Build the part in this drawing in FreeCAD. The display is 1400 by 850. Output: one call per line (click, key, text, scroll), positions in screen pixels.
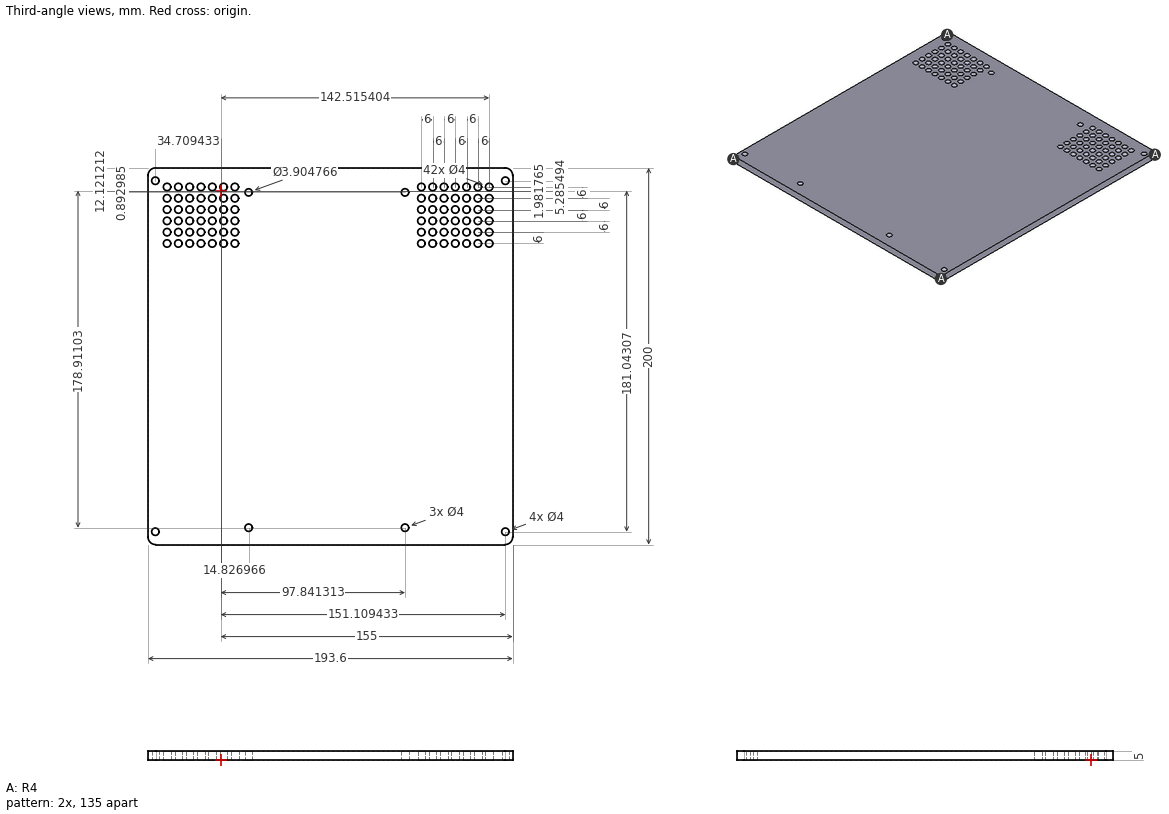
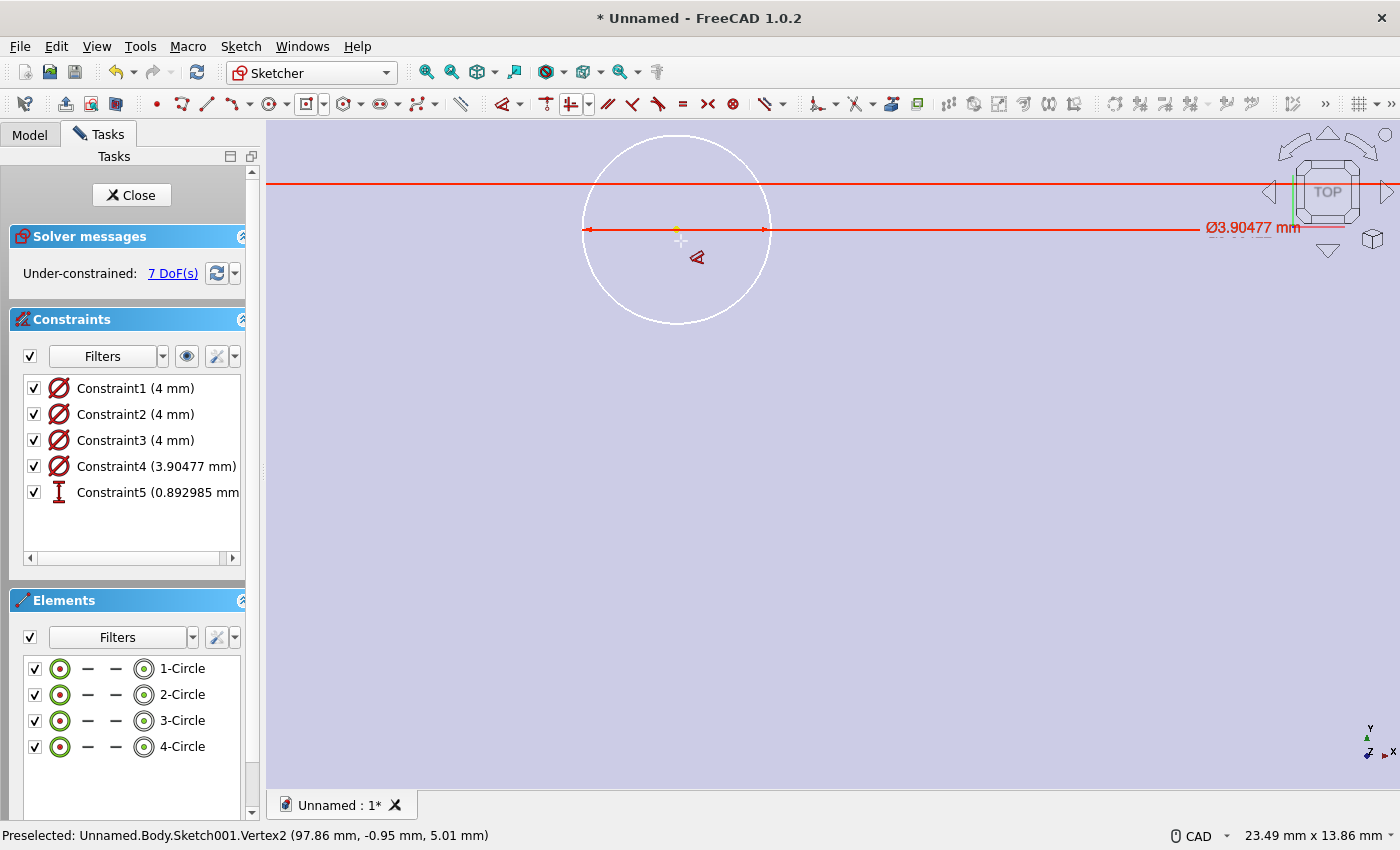
click(677, 230)
click(711, 207)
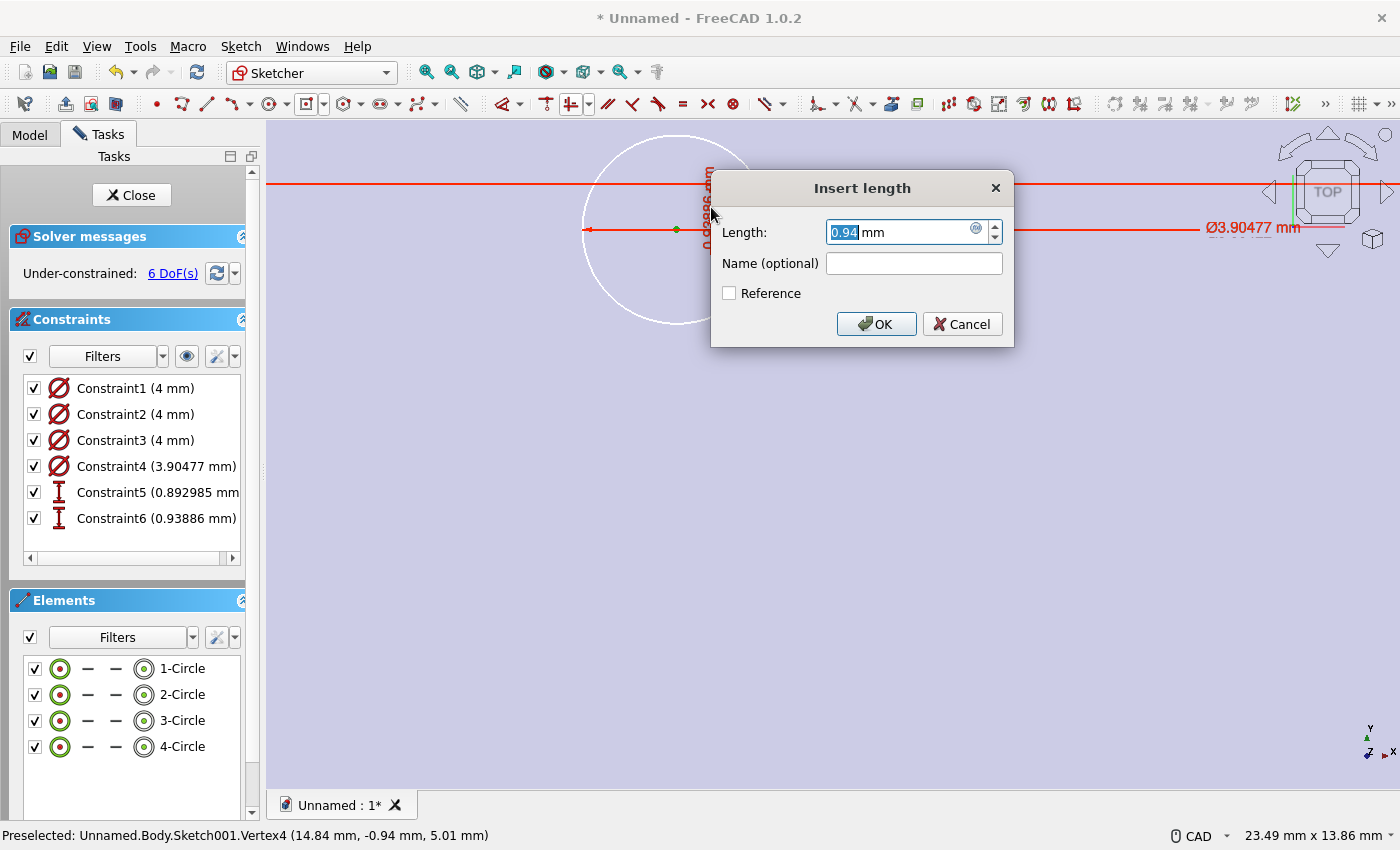
text(0.892985)
key(Return)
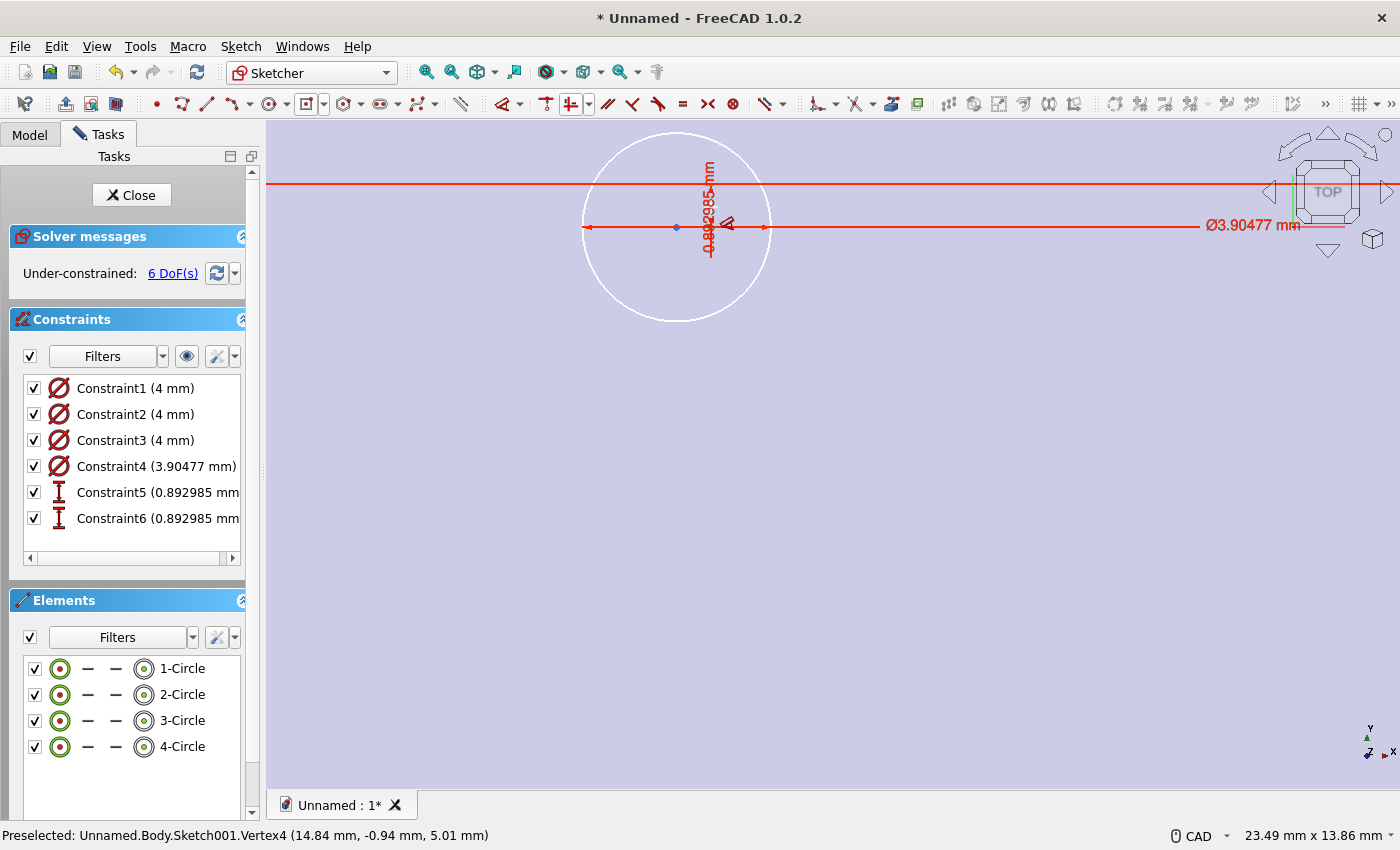
scroll(680, 241, down, 15)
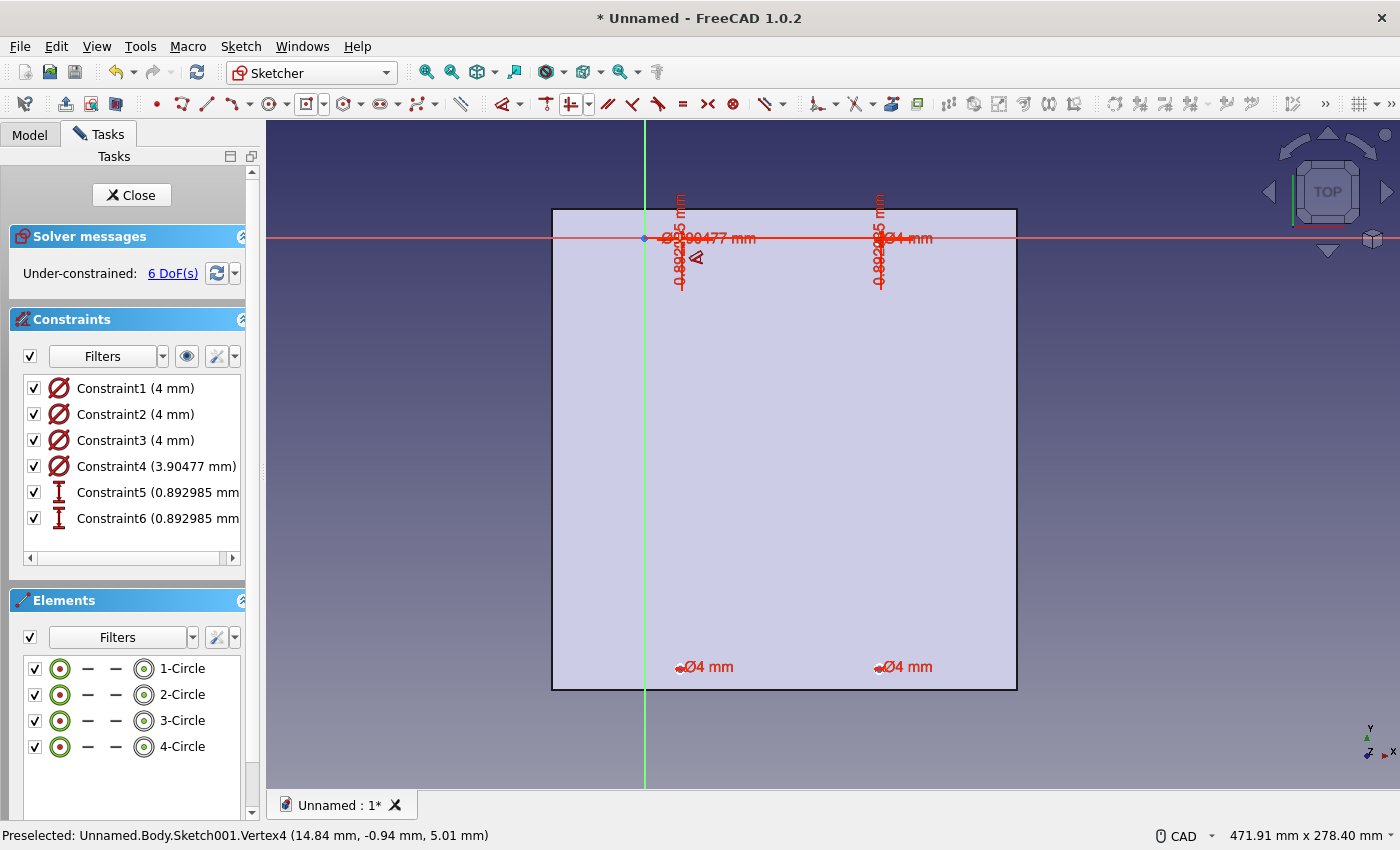
click(879, 669)
click(762, 204)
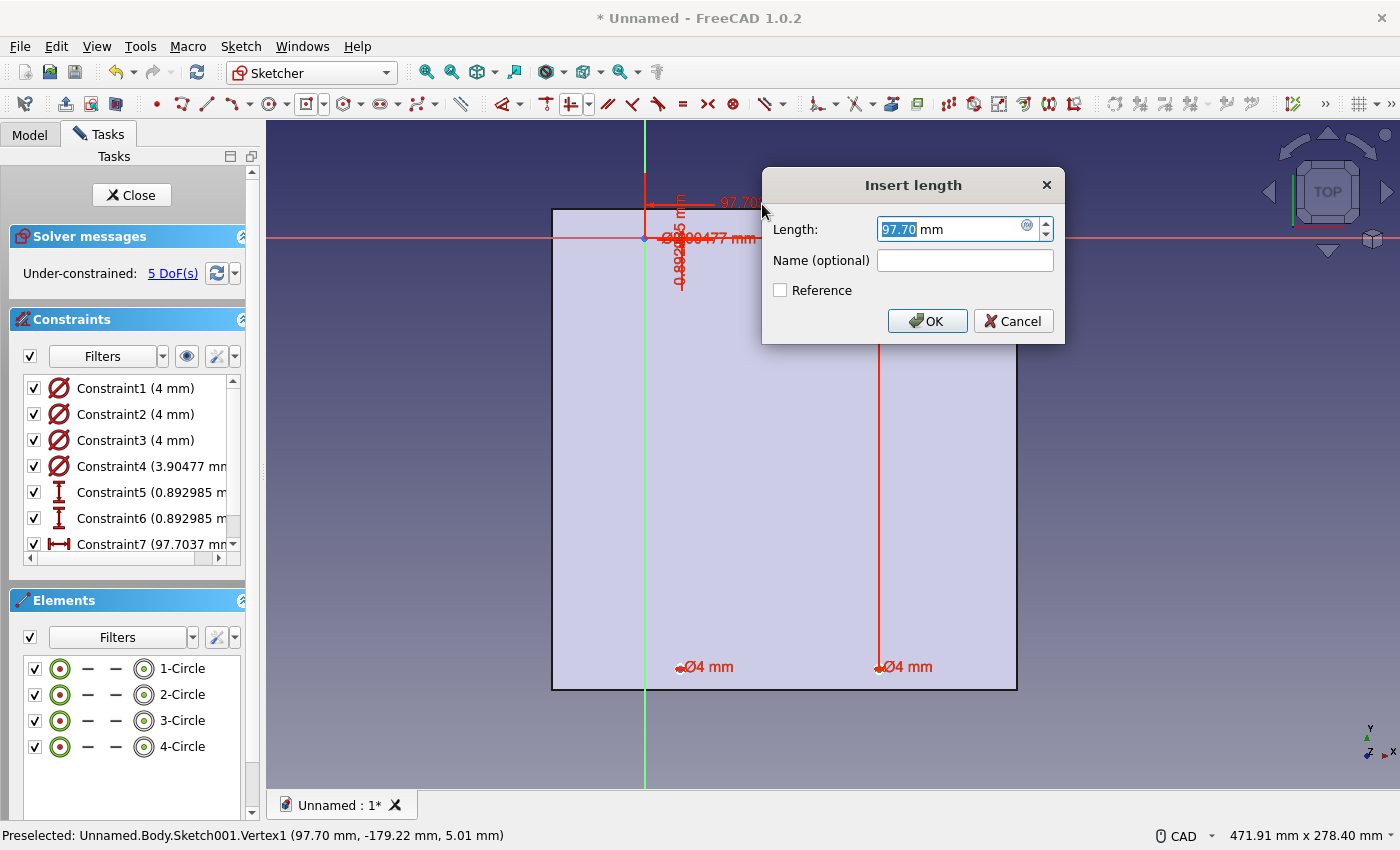
text(97.841313)
key(Return)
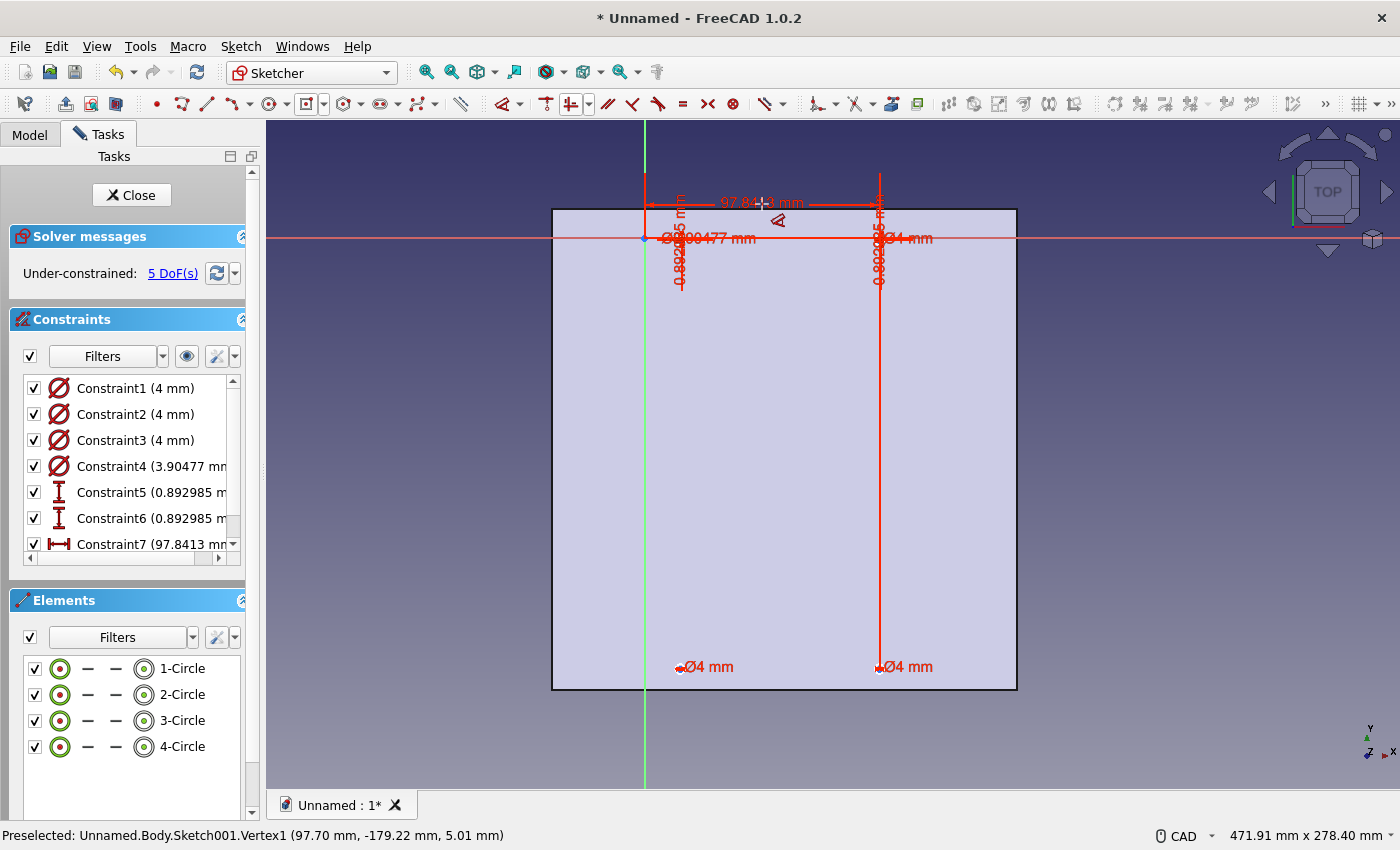
click(880, 669)
click(611, 454)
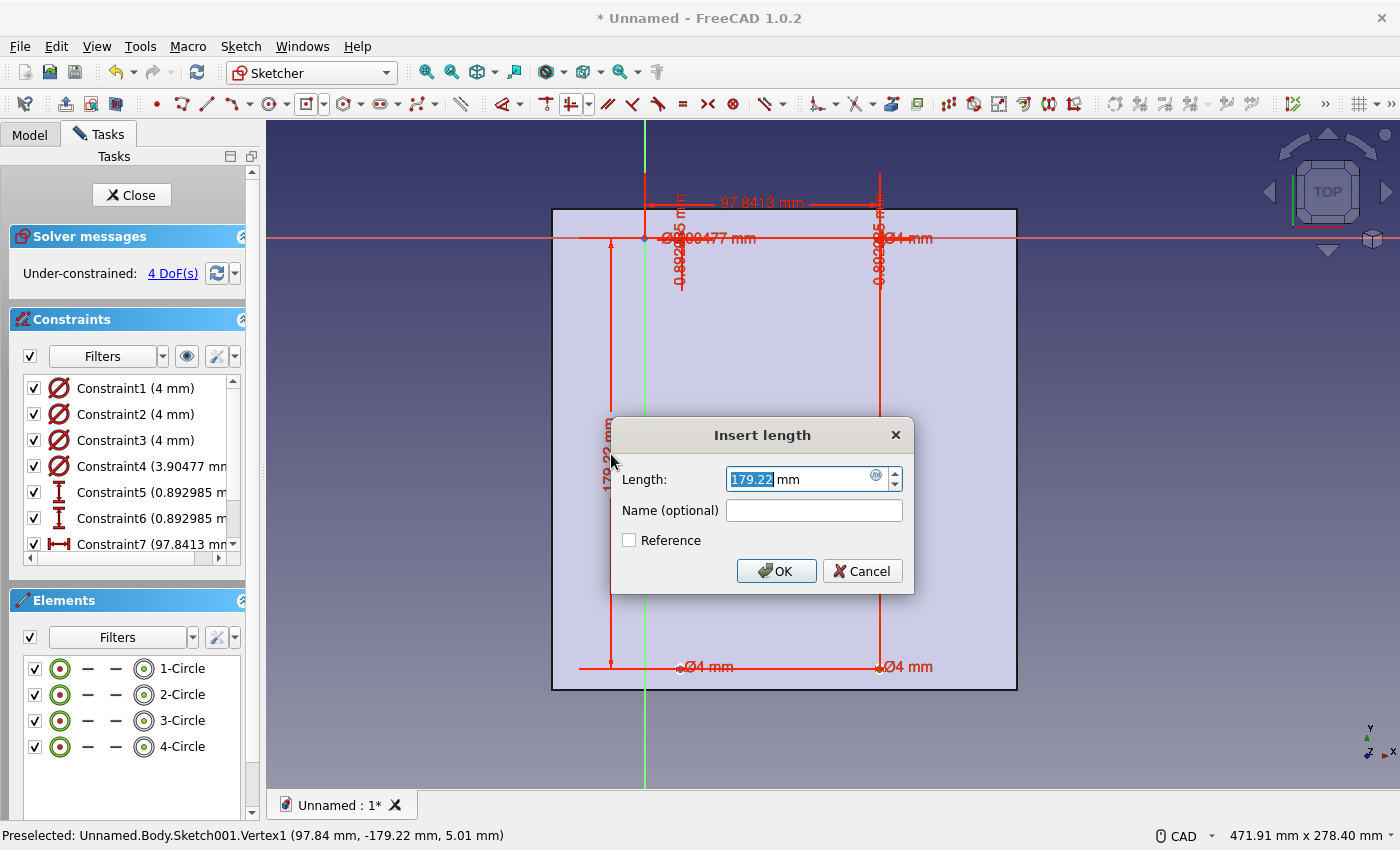
text(178.91103)
key(Return)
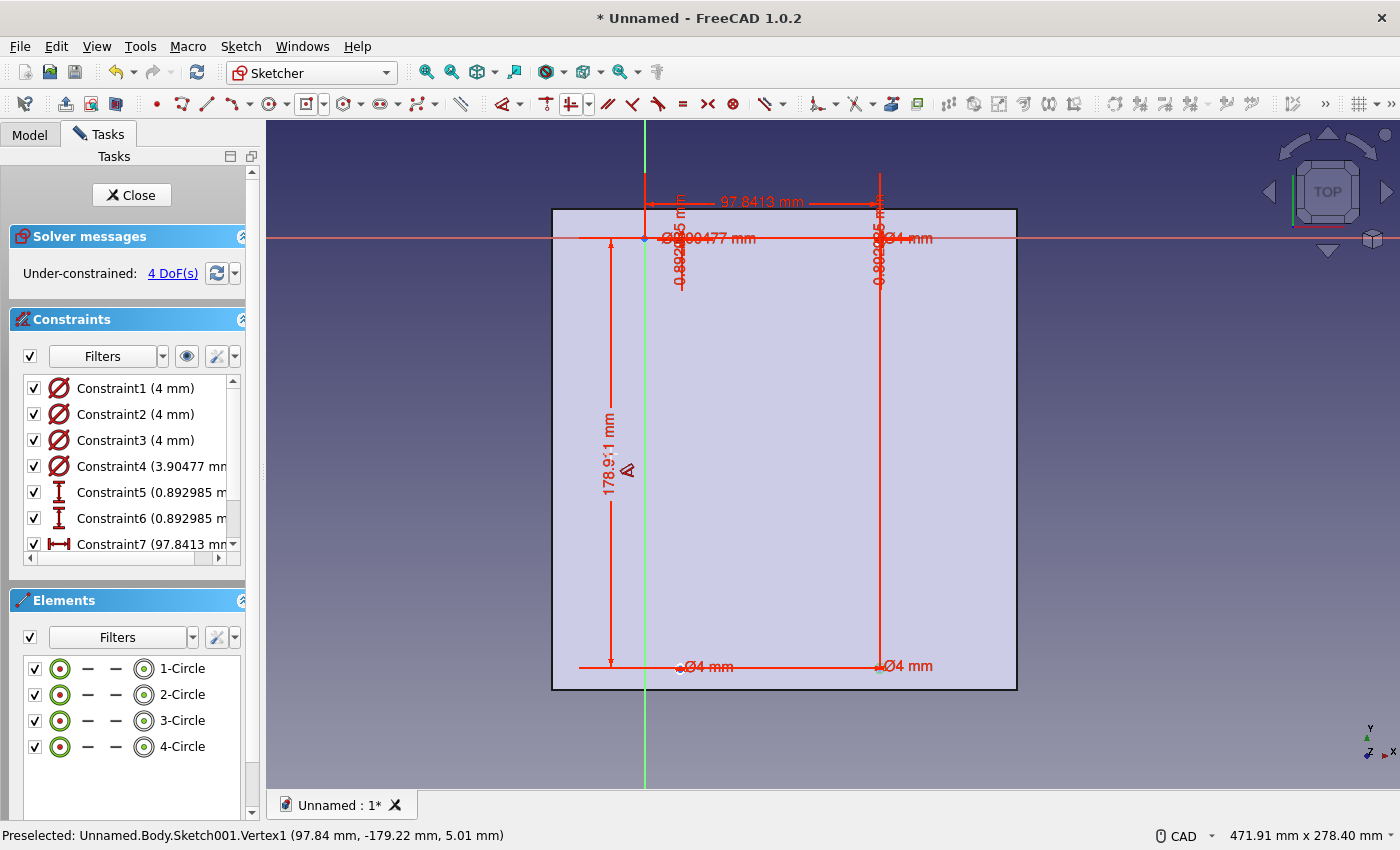
click(880, 240)
click(680, 204)